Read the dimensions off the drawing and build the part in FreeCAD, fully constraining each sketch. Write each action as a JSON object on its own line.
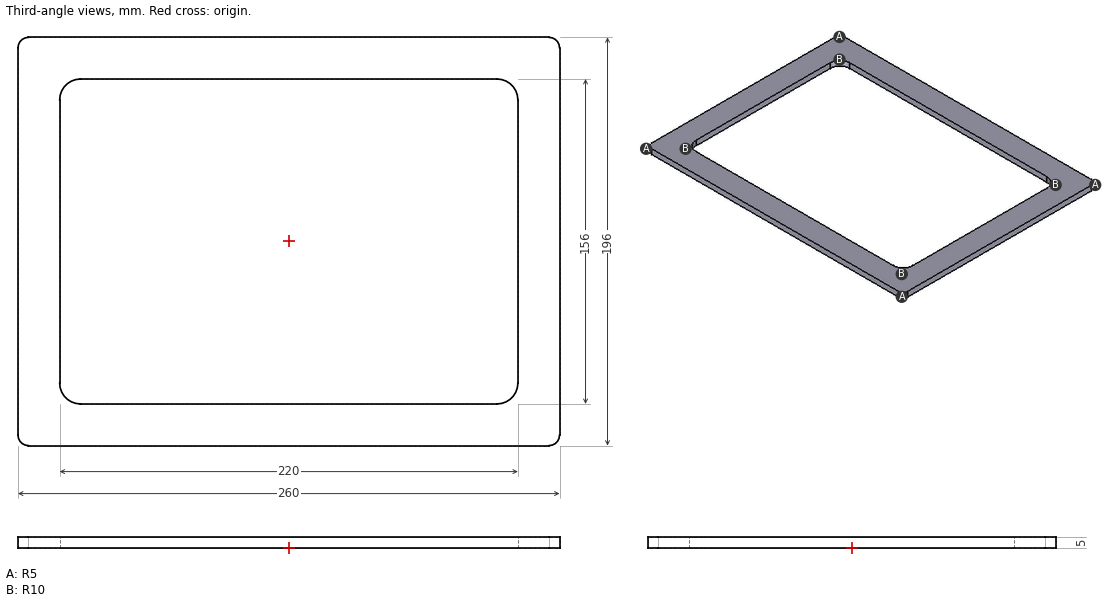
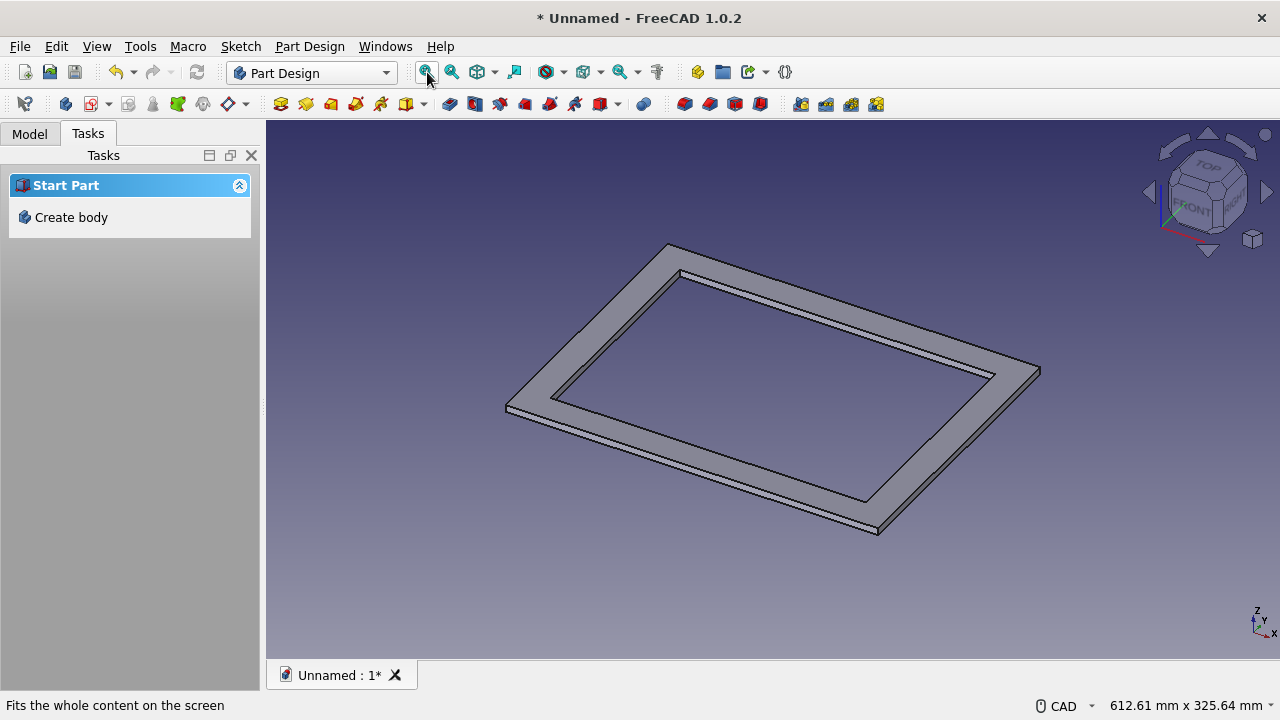
{"action": "scroll", "coordinate": [668, 246], "scroll_direction": "up", "scroll_amount": 8}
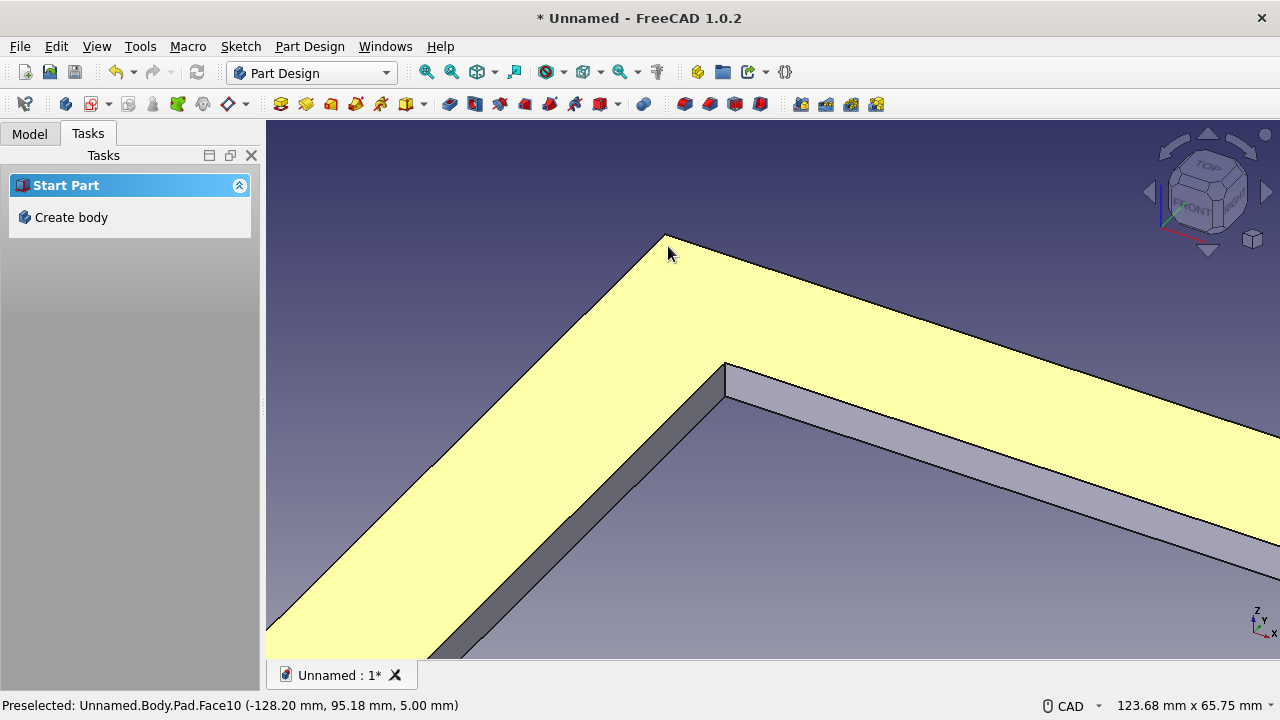
{"action": "left_click", "coordinate": [427, 72]}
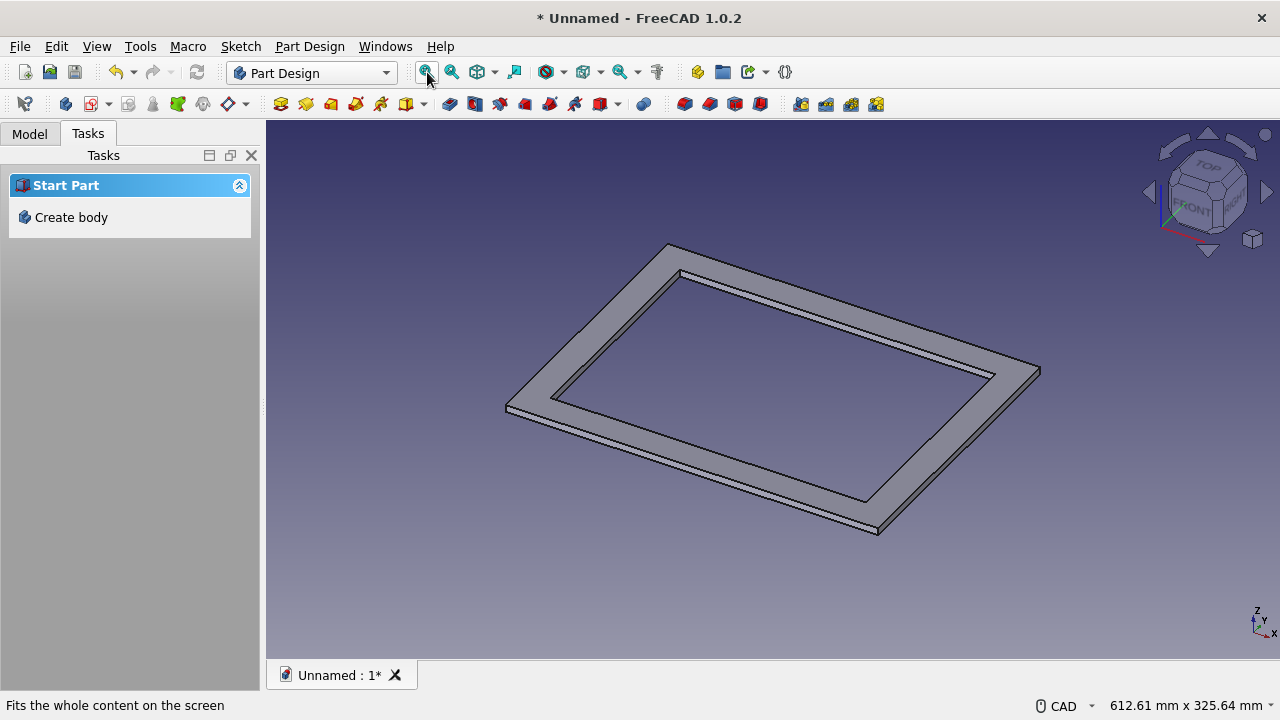
{"action": "key", "text": "0"}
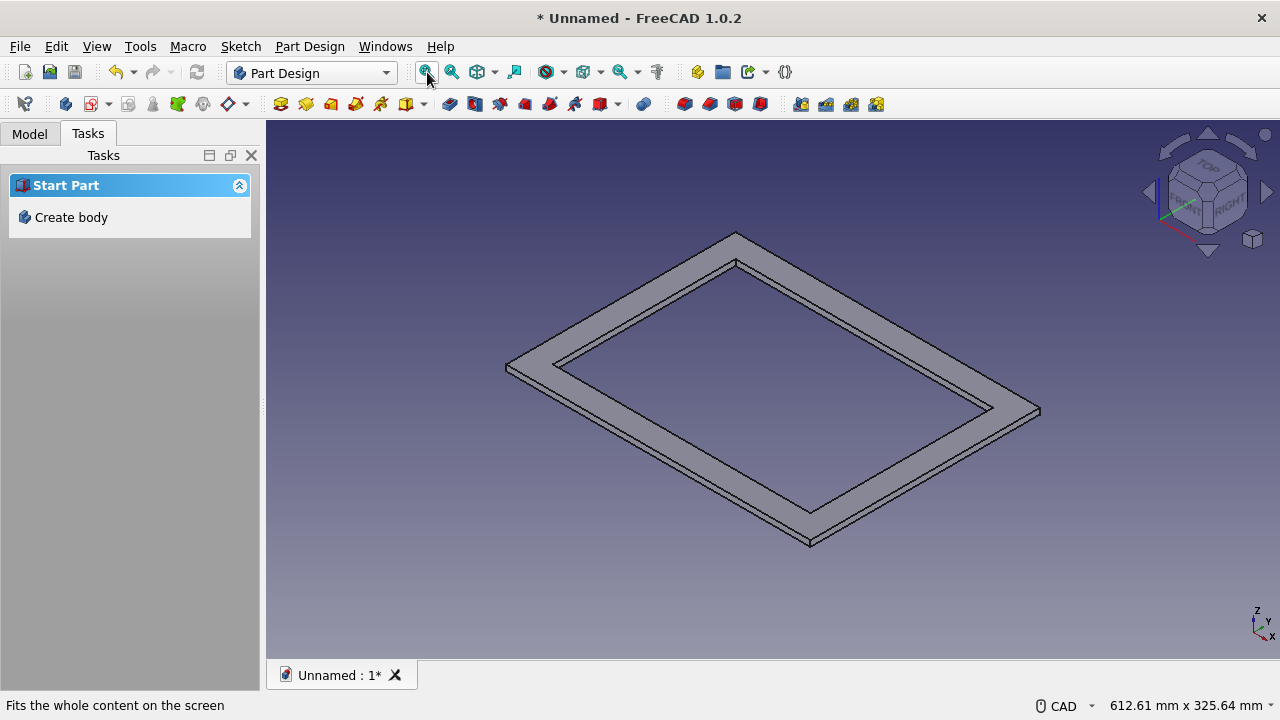
{"action": "scroll", "coordinate": [736, 234], "scroll_direction": "up", "scroll_amount": 8}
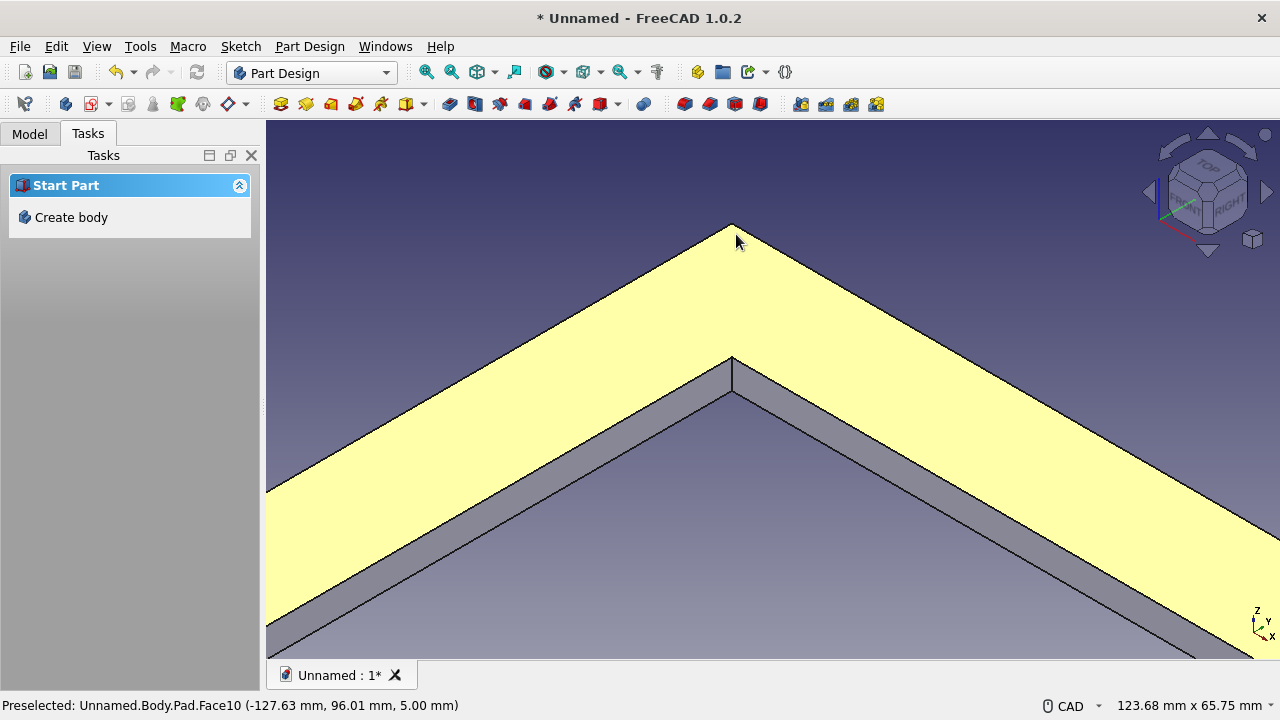
{"action": "left_click", "coordinate": [427, 72]}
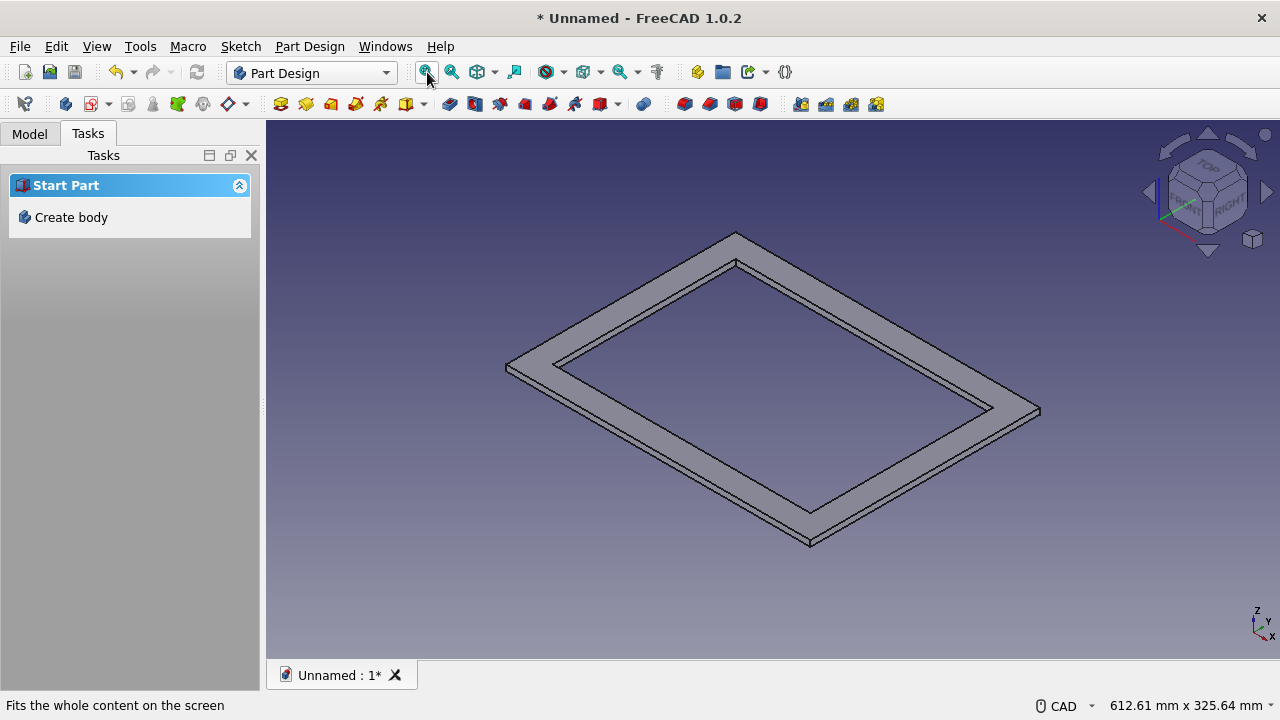
{"action": "key", "text": "2"}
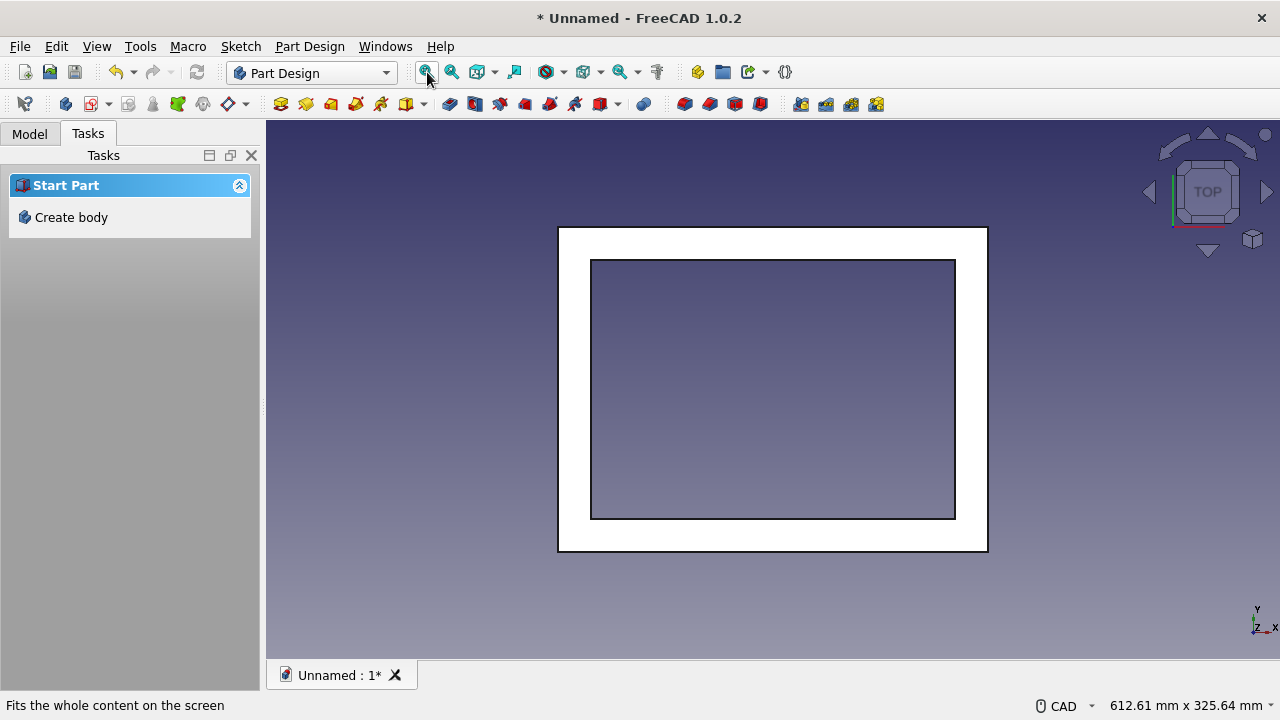
{"action": "scroll", "coordinate": [558, 226], "scroll_direction": "up", "scroll_amount": 8}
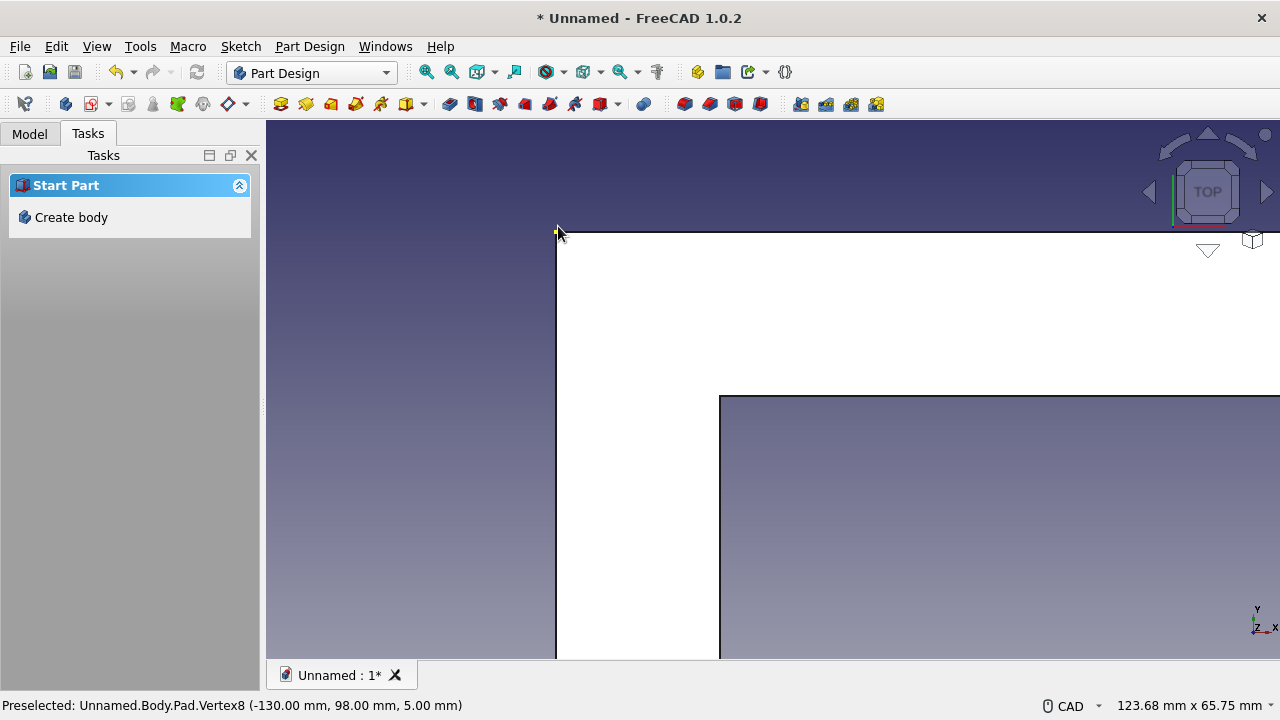
{"action": "key", "text": "v f"}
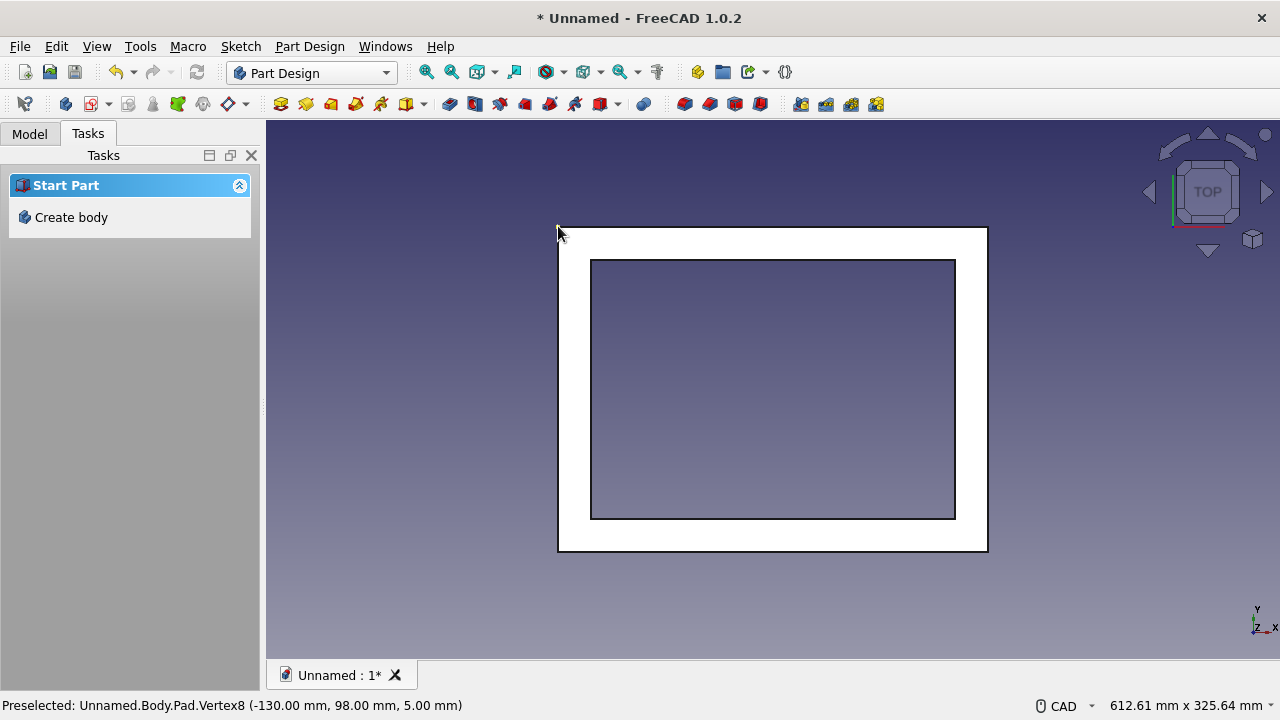
{"action": "key", "text": "1"}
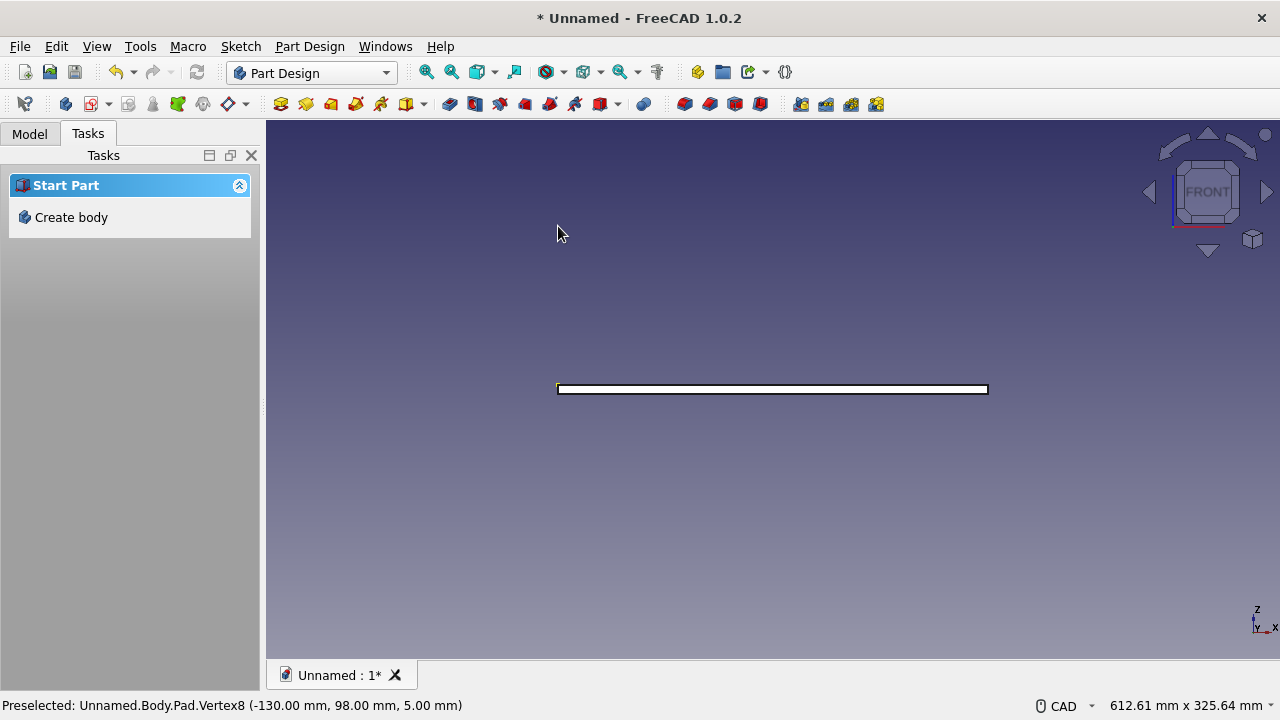
{"action": "left_click", "coordinate": [427, 72]}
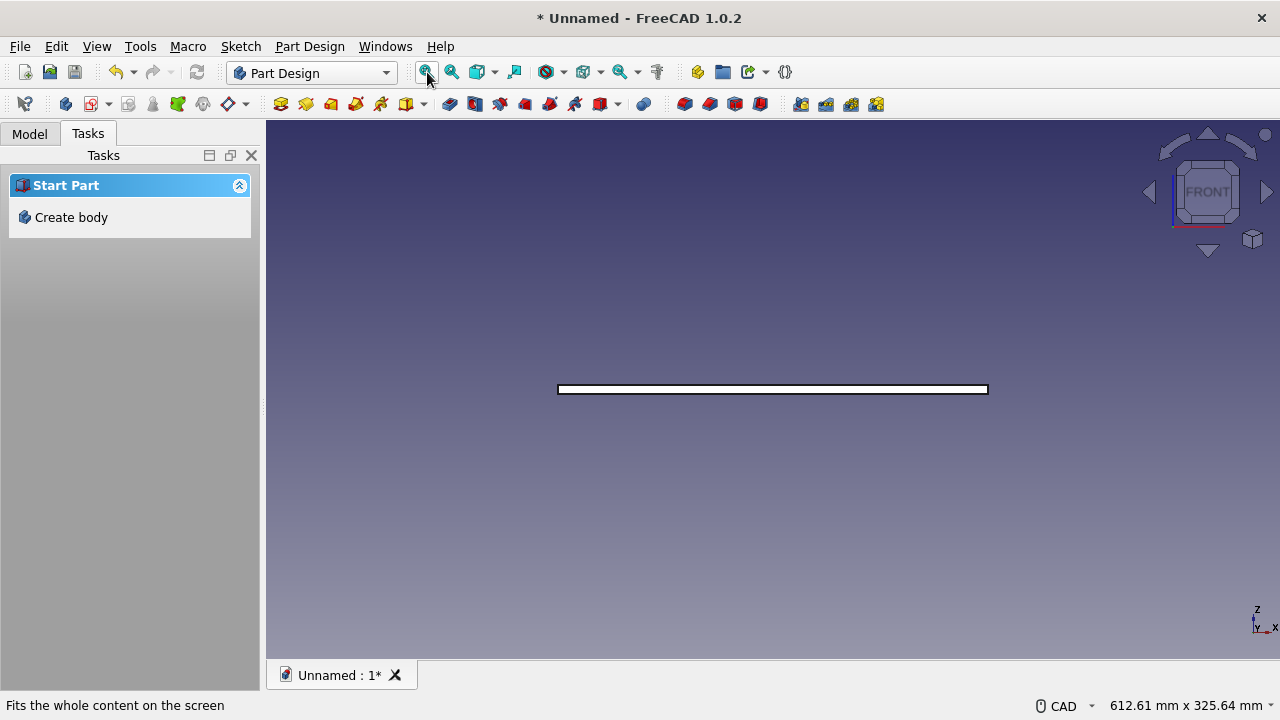
{"action": "scroll", "coordinate": [558, 389], "scroll_direction": "up", "scroll_amount": 8}